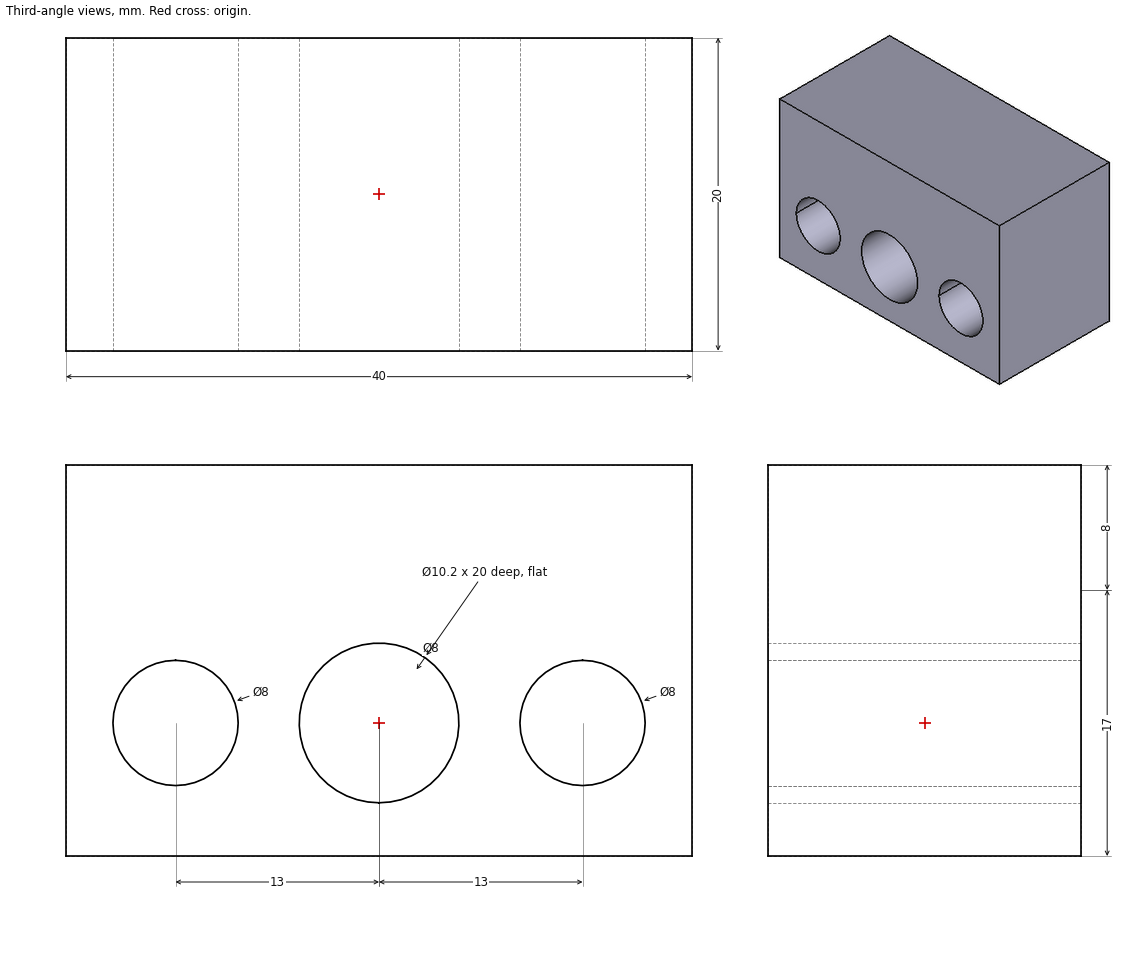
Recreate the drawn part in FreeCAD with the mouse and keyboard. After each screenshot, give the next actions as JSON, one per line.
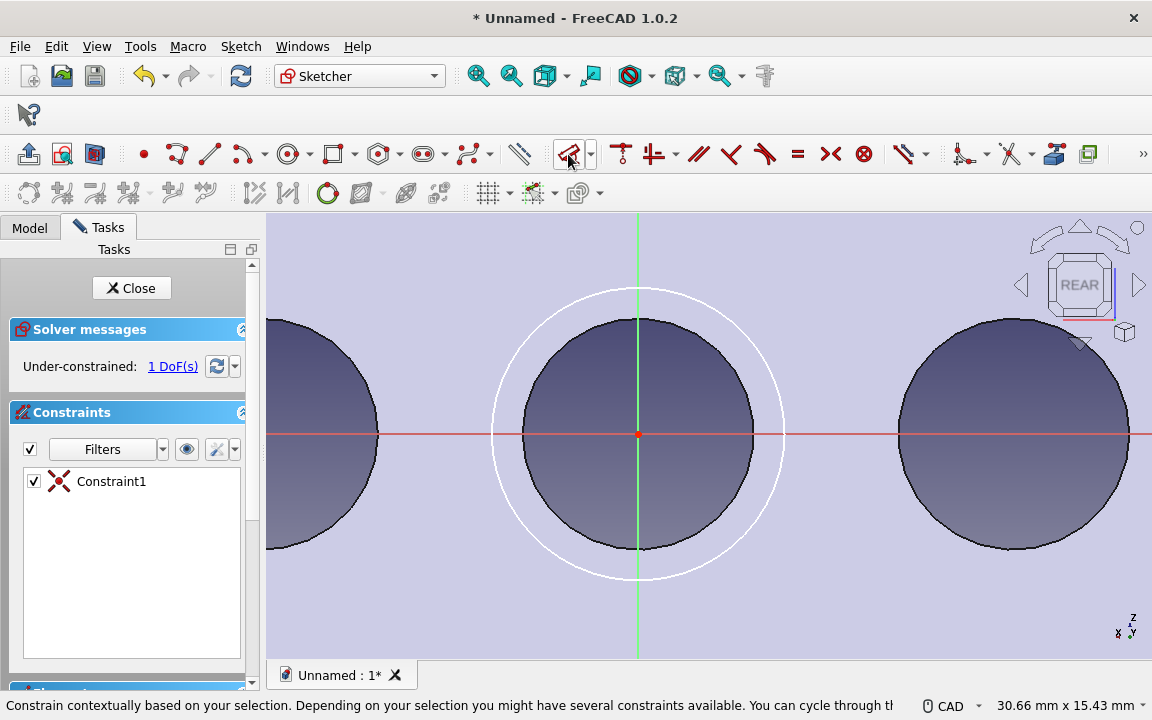
{"action": "left_click", "coordinate": [741, 330]}
{"action": "left_click", "coordinate": [763, 307]}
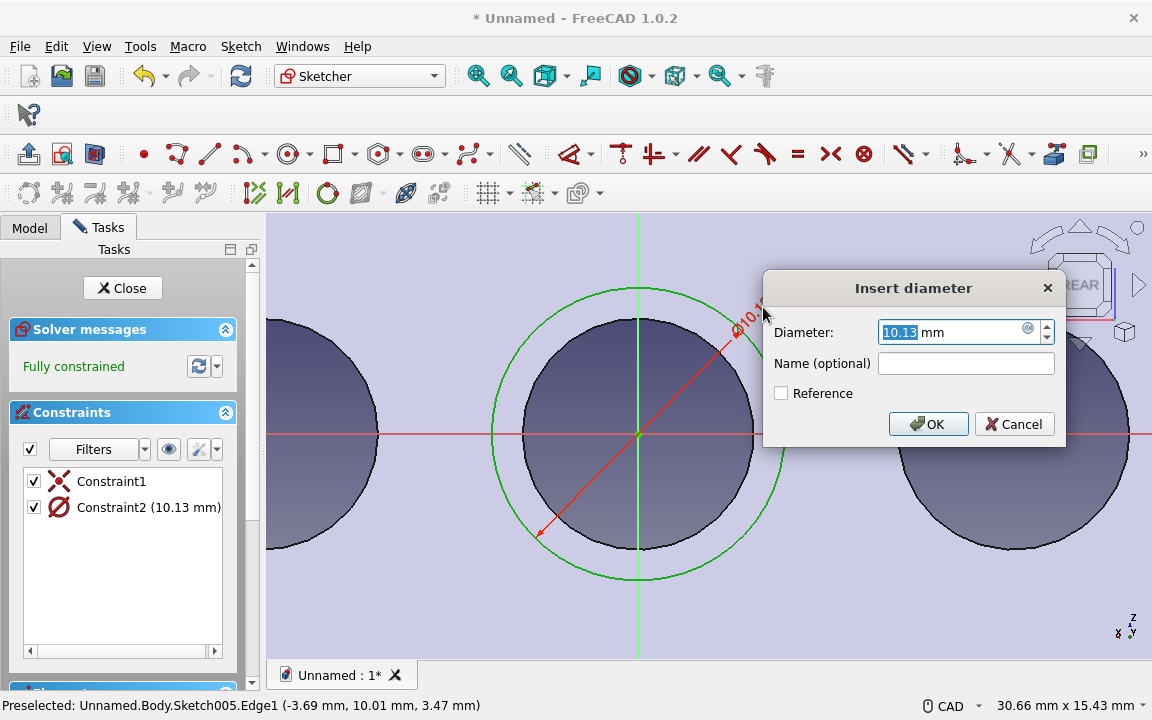
{"action": "type", "text": "10.2"}
{"action": "key", "text": "Return"}
{"action": "key", "text": "Escape"}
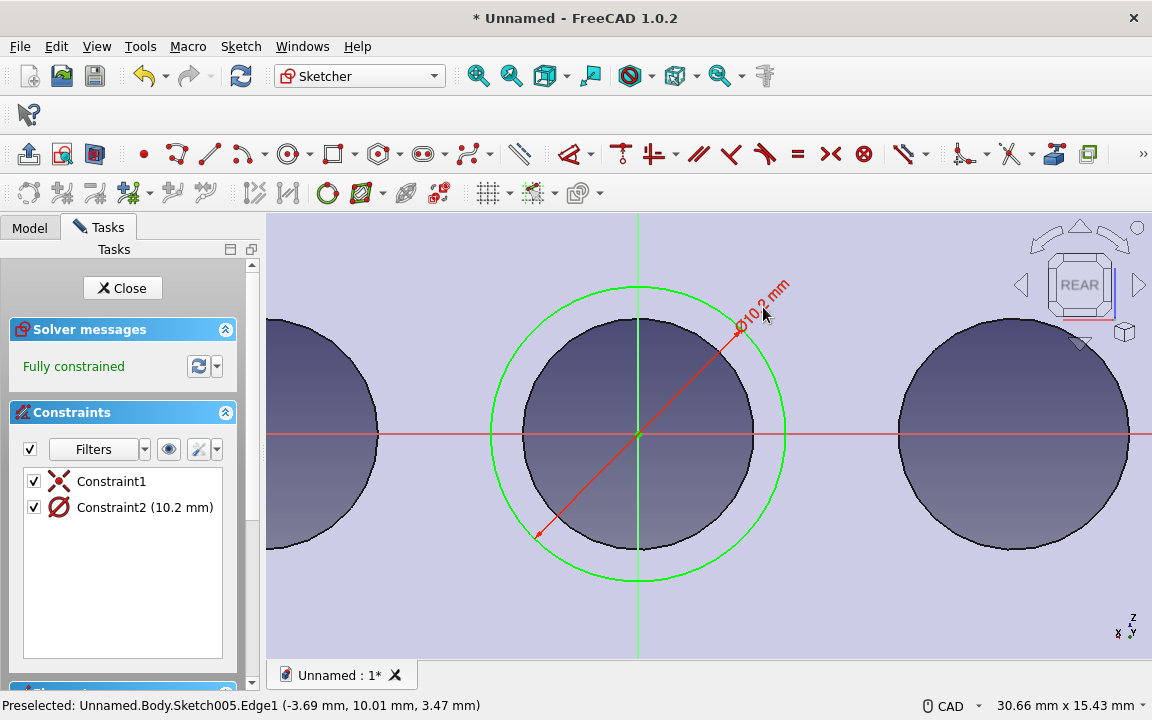
{"action": "left_click", "coordinate": [123, 288]}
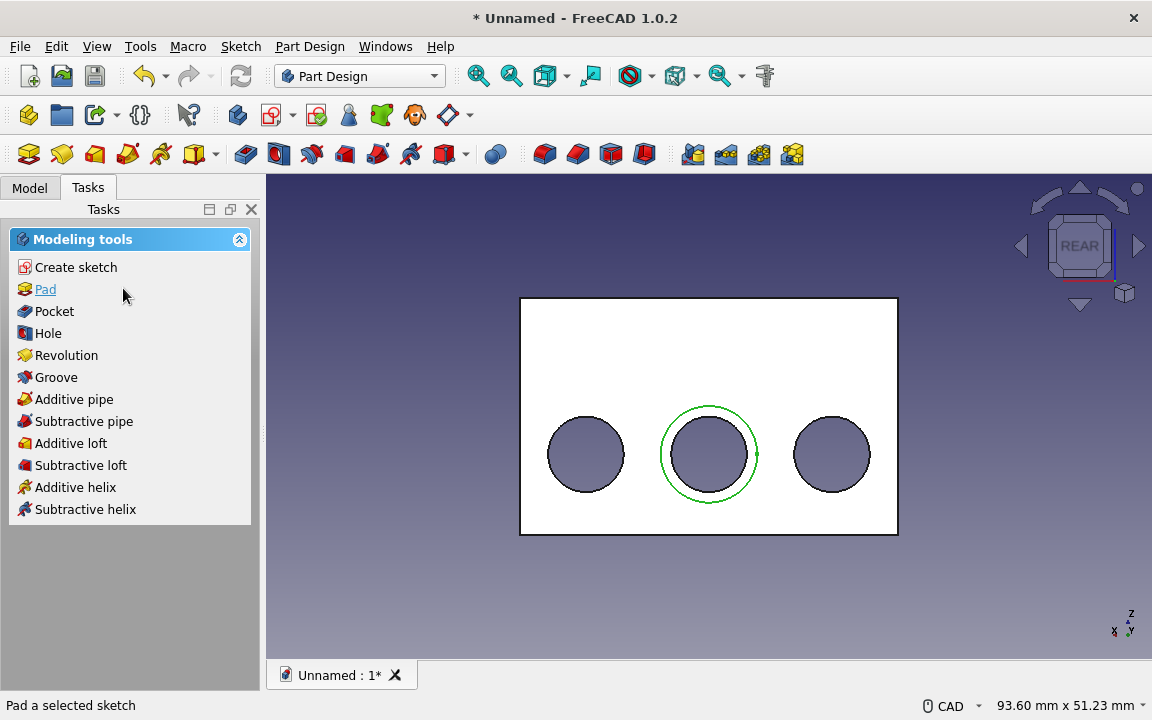
{"action": "left_click", "coordinate": [279, 154]}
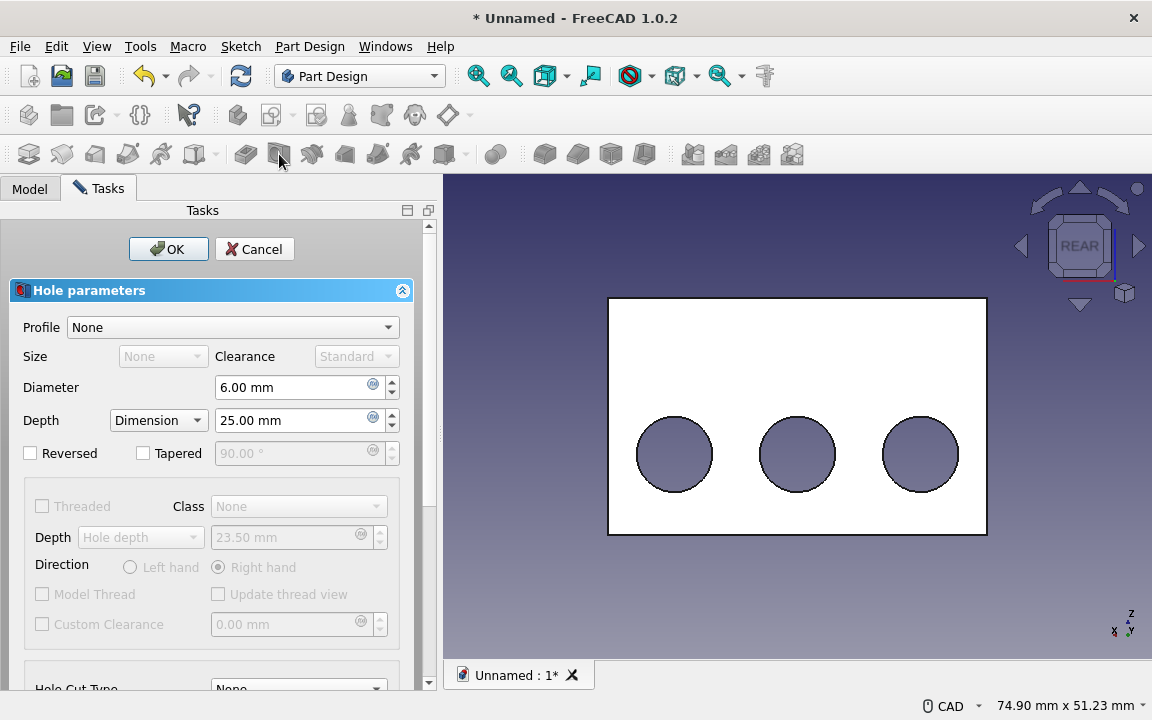
{"action": "triple_click", "coordinate": [300, 388]}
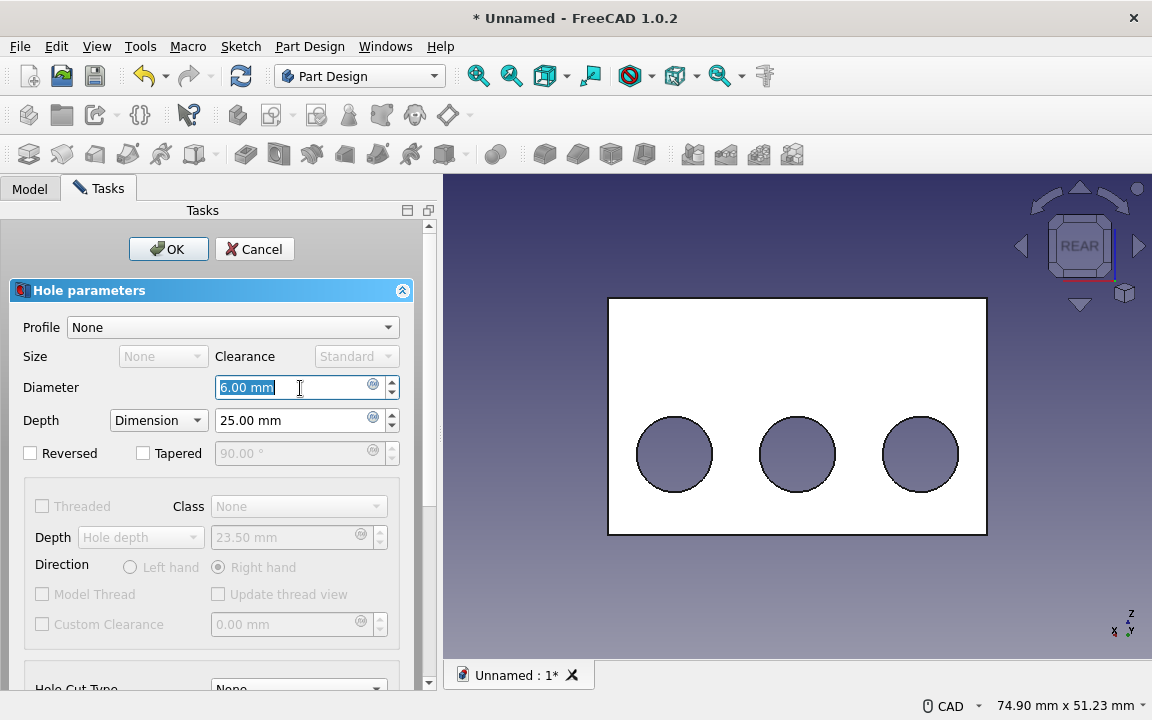
{"action": "type", "text": "10.2"}
{"action": "key", "text": "Tab"}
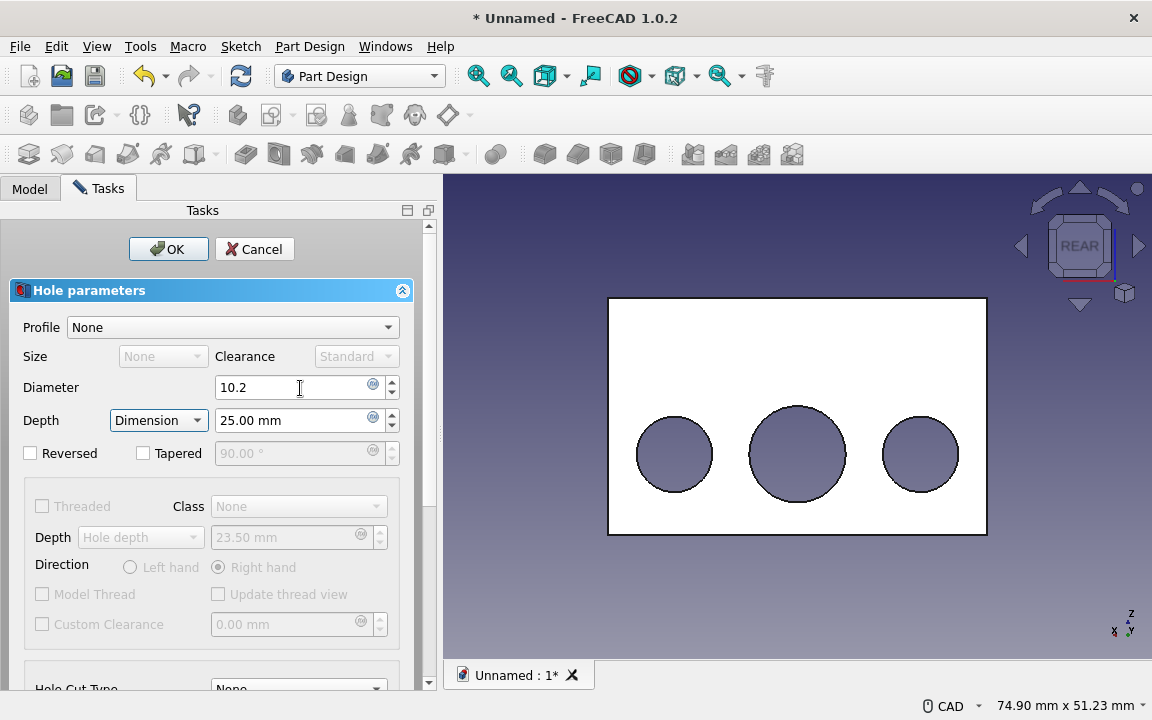
{"action": "triple_click", "coordinate": [300, 420]}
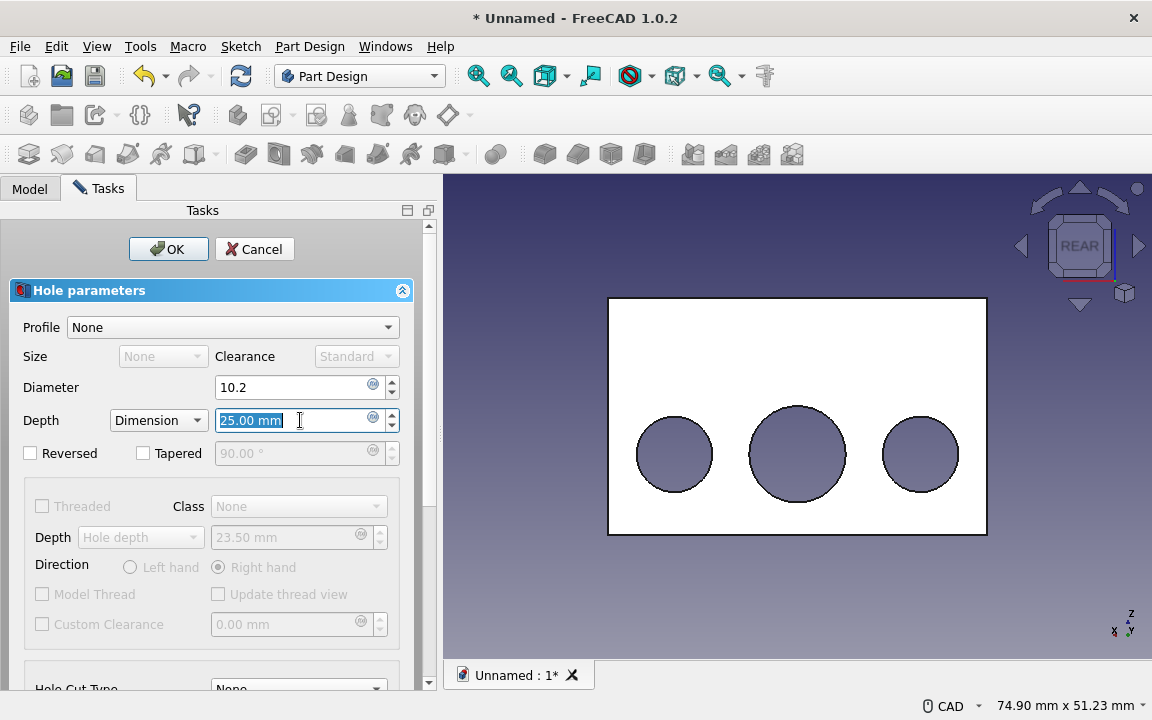
{"action": "type", "text": "20"}
{"action": "key", "text": "Tab"}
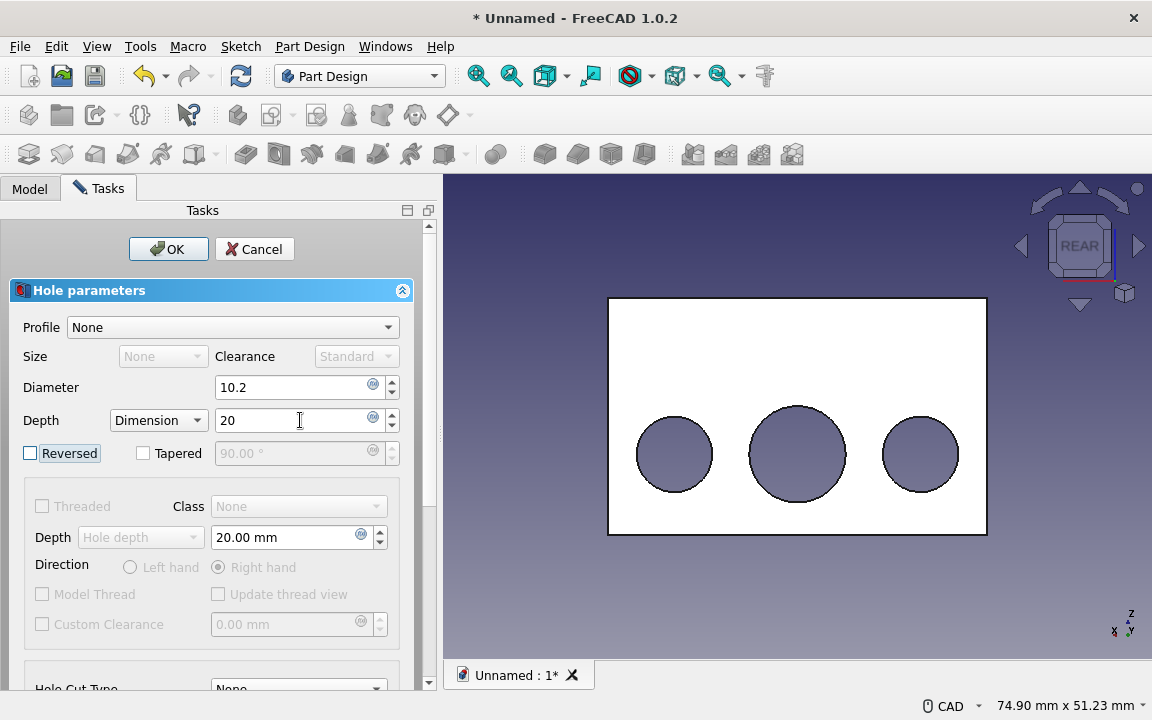
{"action": "scroll", "coordinate": [429, 455], "scroll_direction": "down", "scroll_amount": 5}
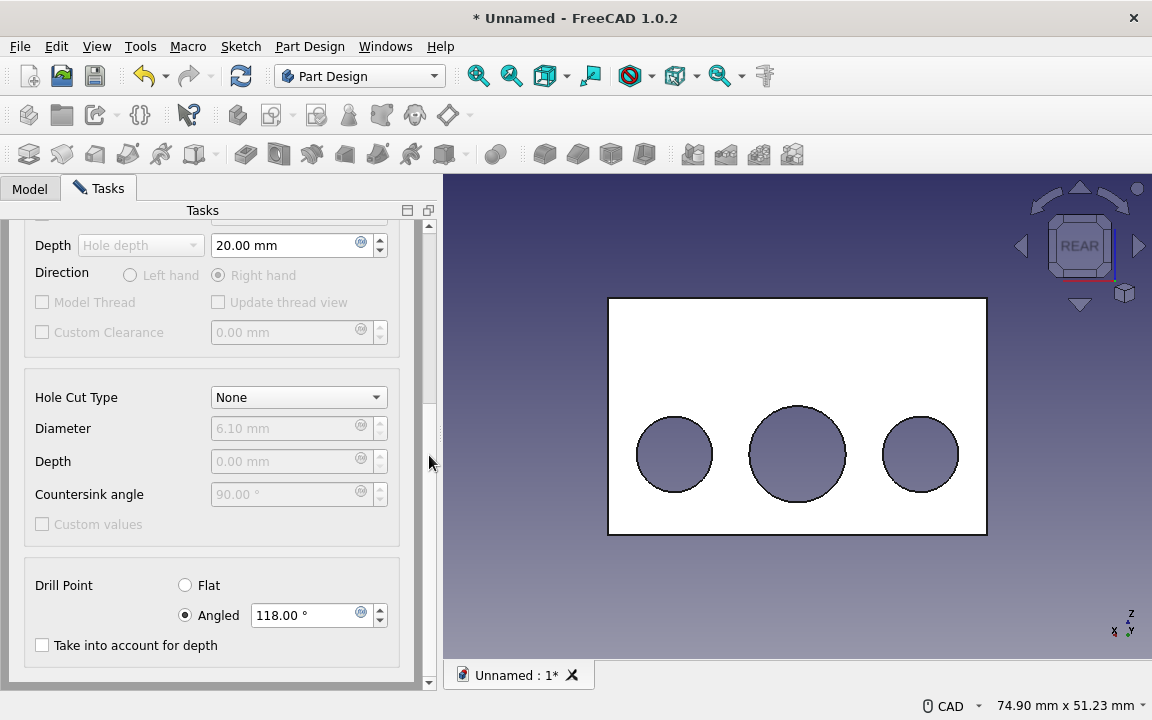
{"action": "left_click", "coordinate": [186, 583]}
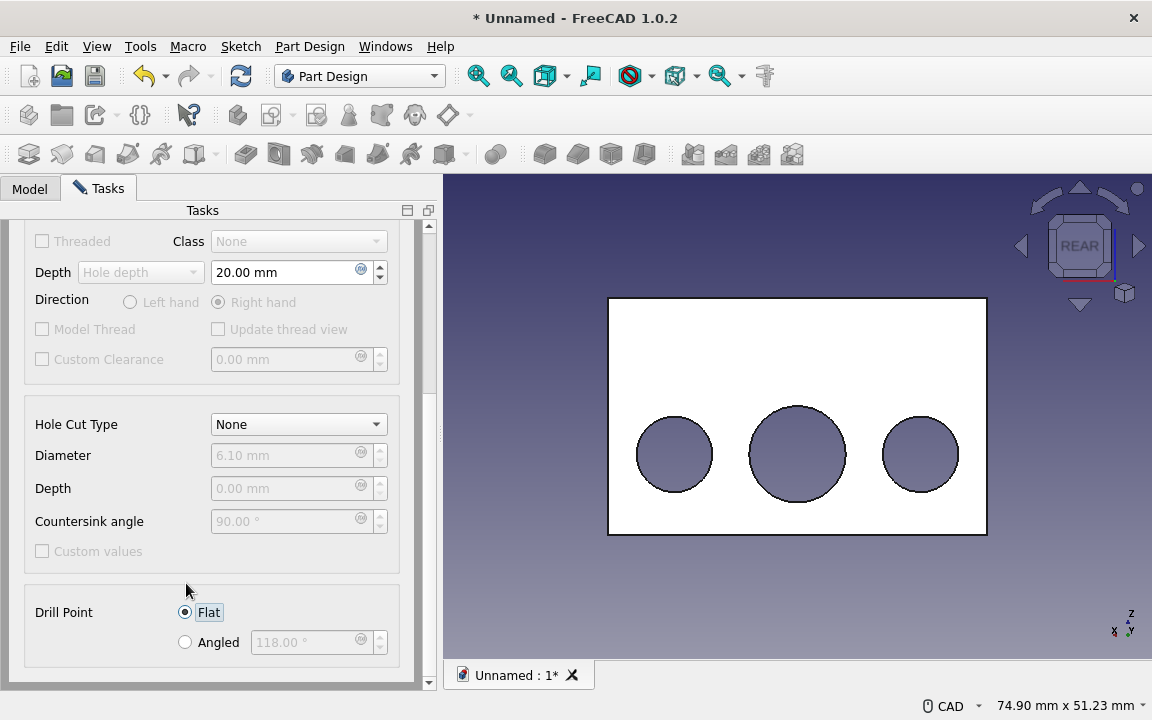
{"action": "scroll", "coordinate": [429, 455], "scroll_direction": "up", "scroll_amount": 6}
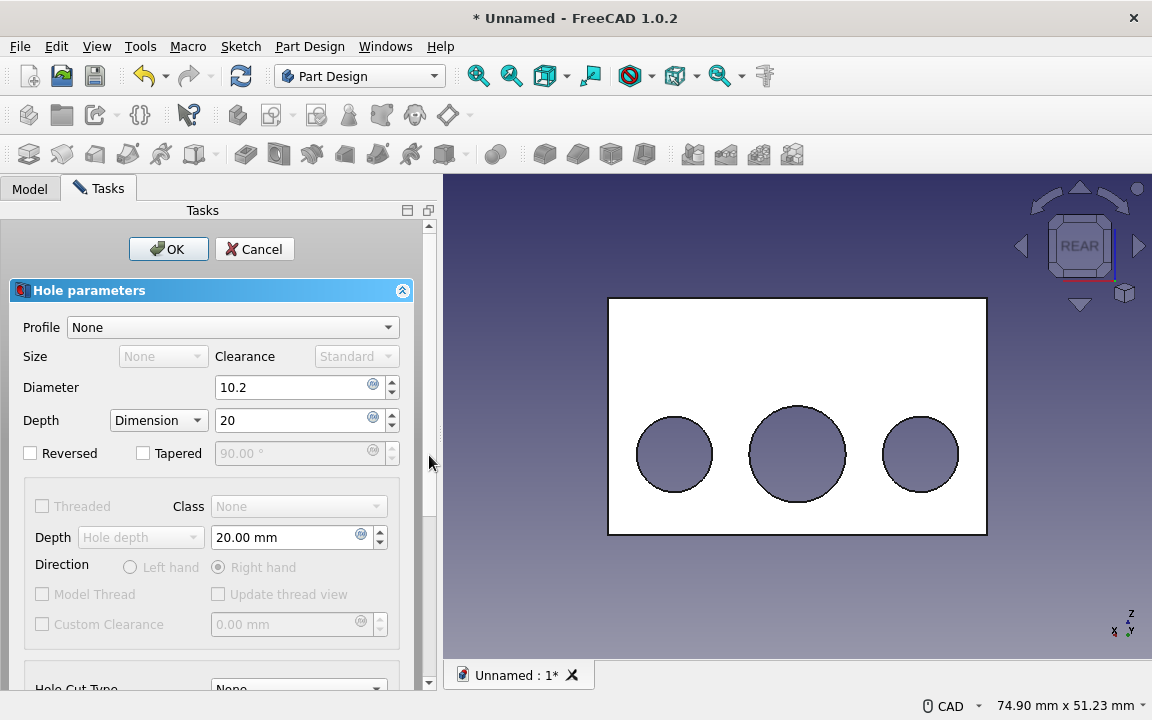
{"action": "left_click", "coordinate": [169, 249]}